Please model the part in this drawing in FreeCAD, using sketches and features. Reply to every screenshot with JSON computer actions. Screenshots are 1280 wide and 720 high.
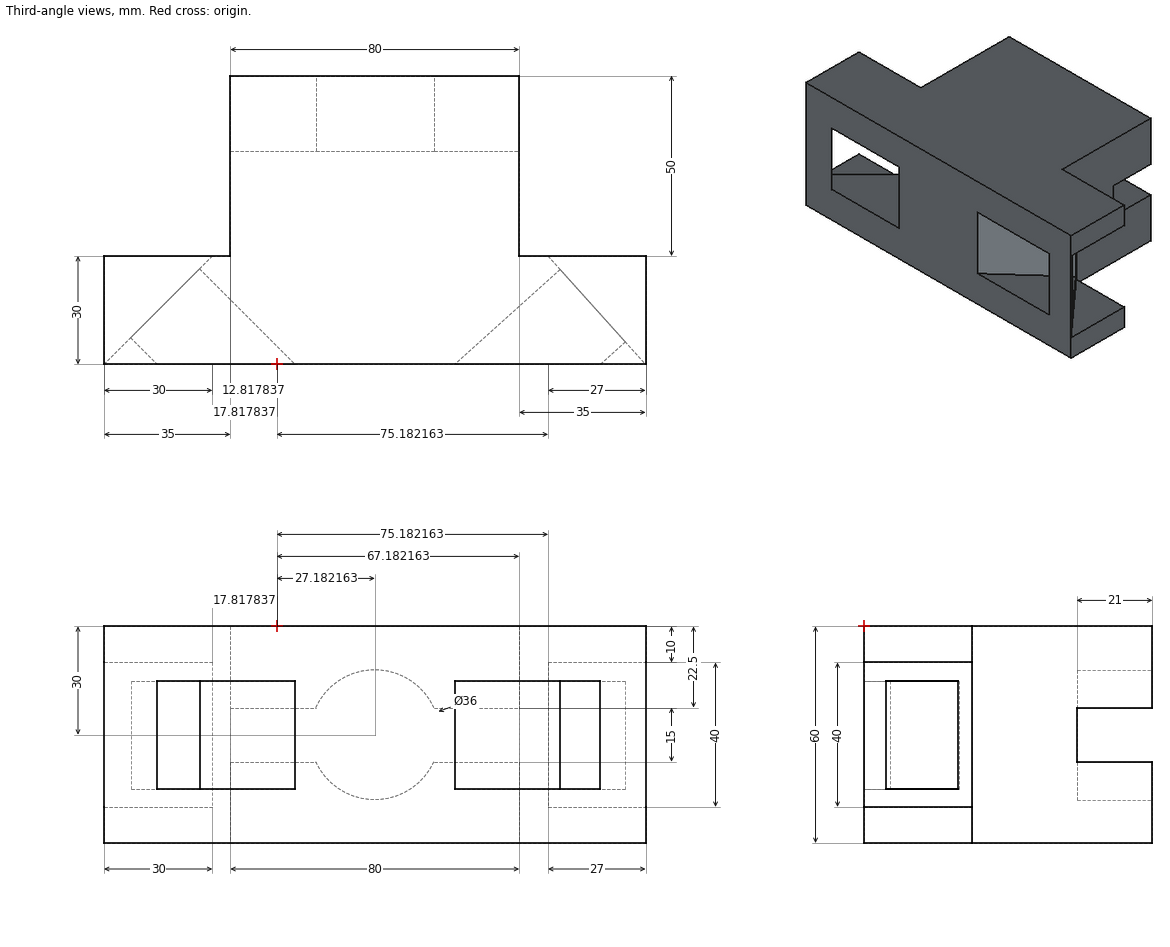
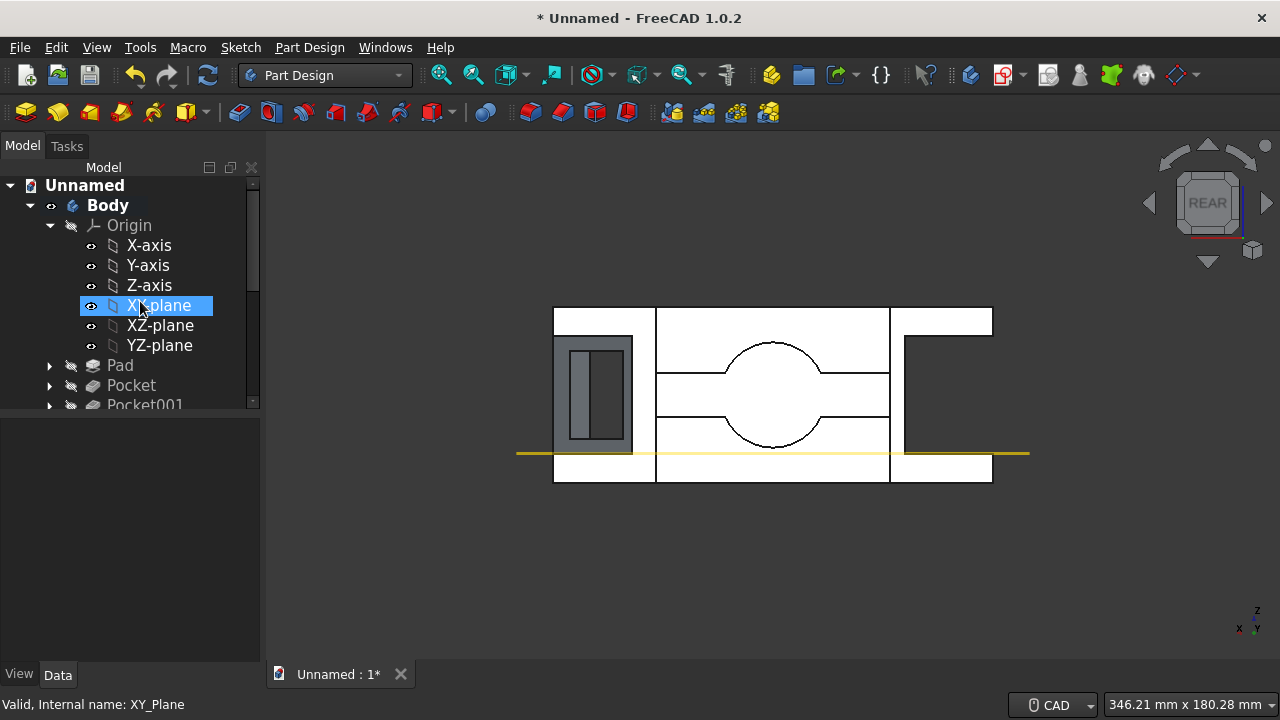
{"action": "scroll", "coordinate": [100, 301], "scroll_direction": "down", "scroll_amount": 6}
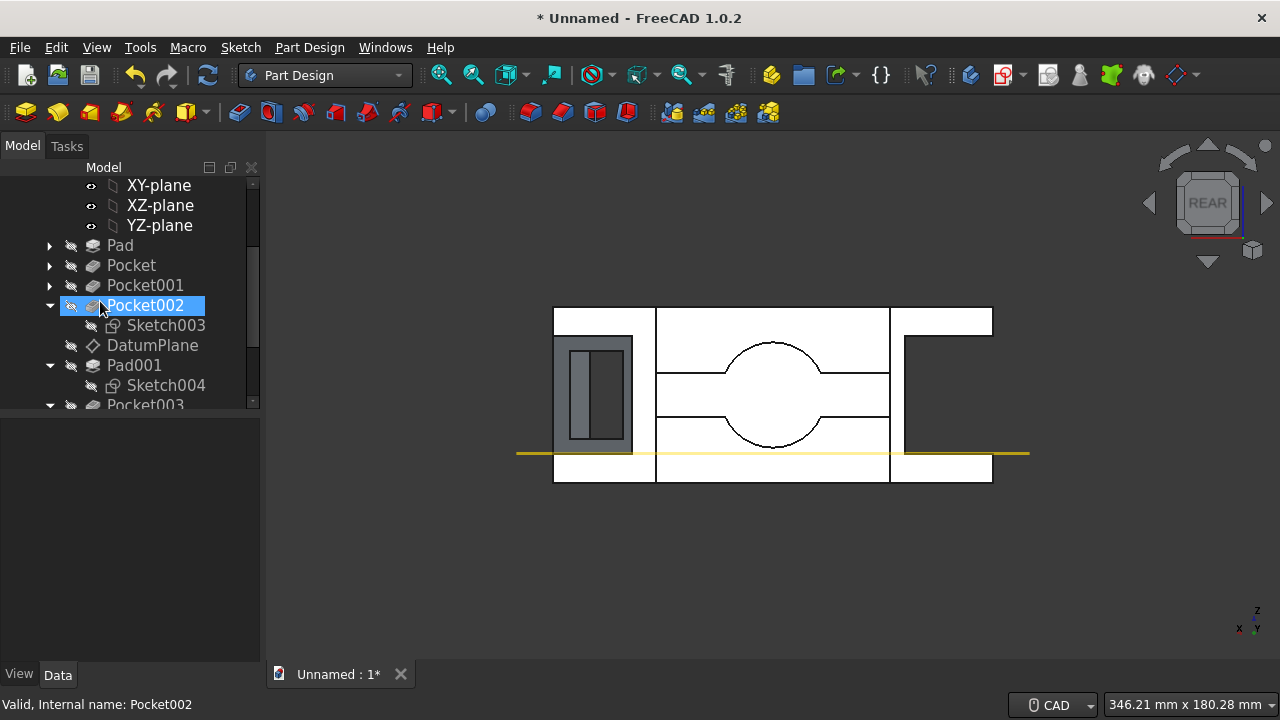
{"action": "left_click", "coordinate": [116, 386]}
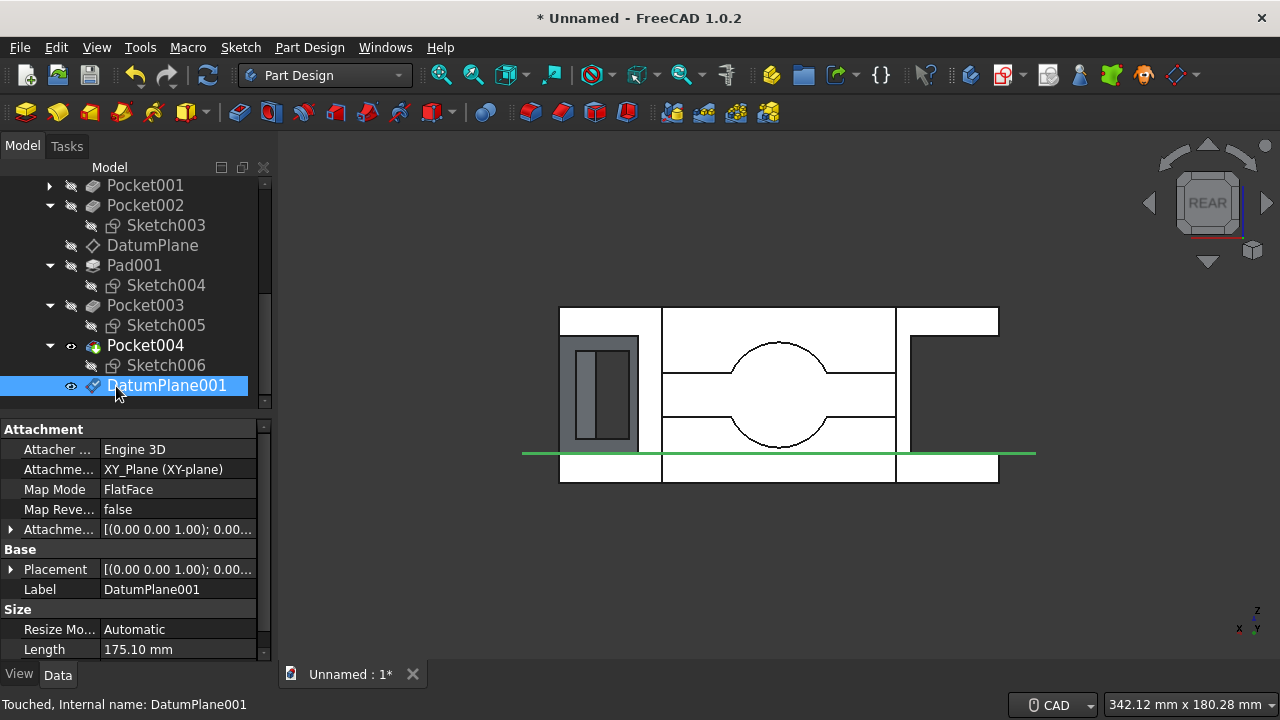
{"action": "left_click", "coordinate": [1004, 76]}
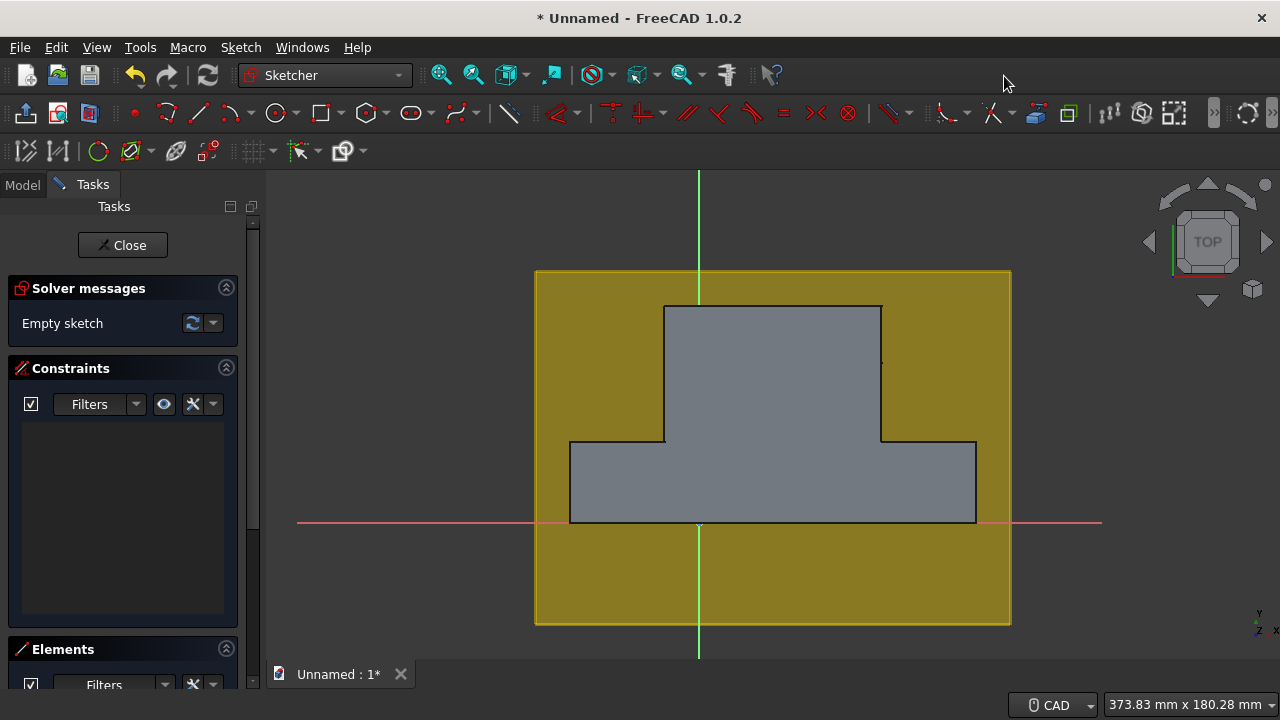
{"action": "left_click", "coordinate": [90, 114]}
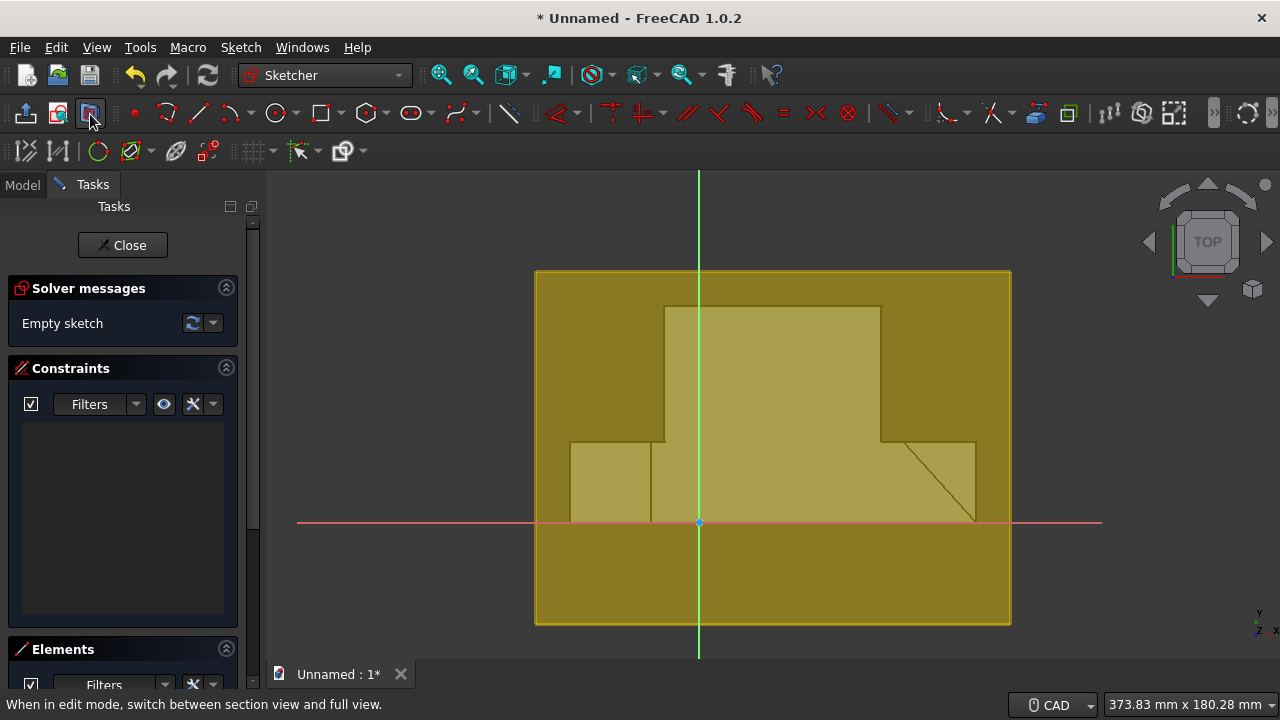
{"action": "scroll", "coordinate": [611, 505], "scroll_direction": "up", "scroll_amount": 7}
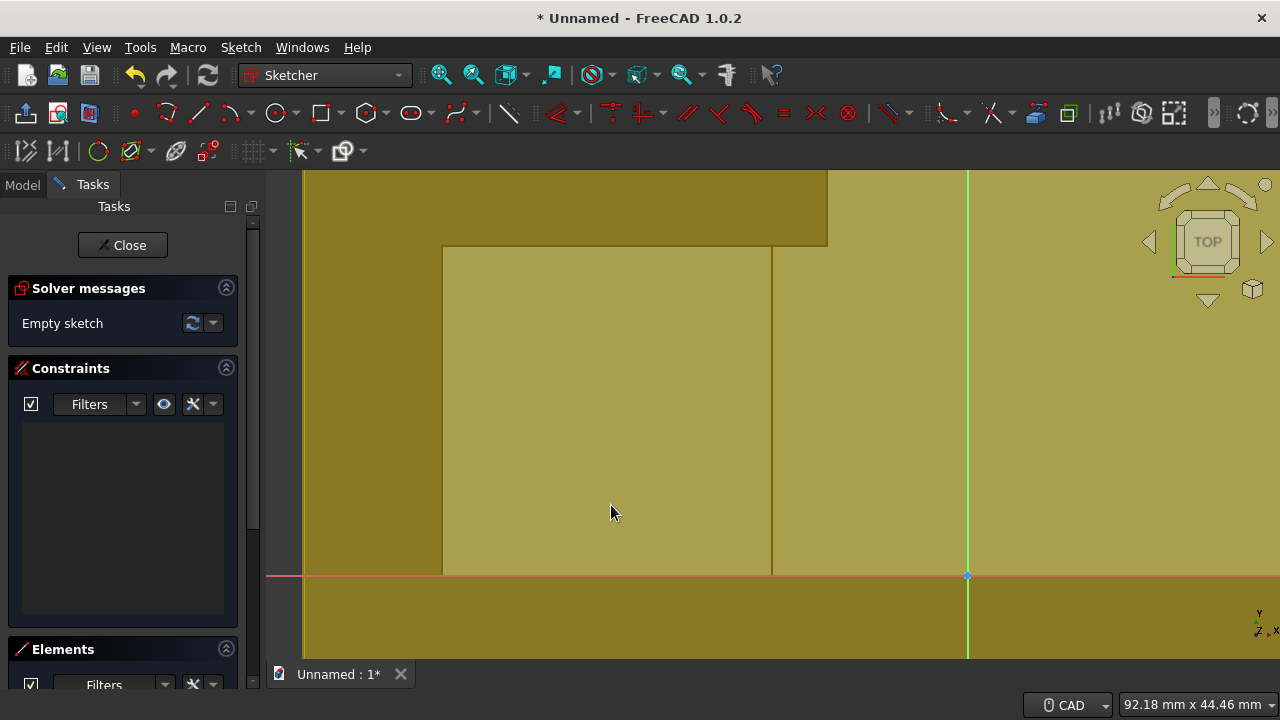
{"action": "left_click", "coordinate": [168, 114]}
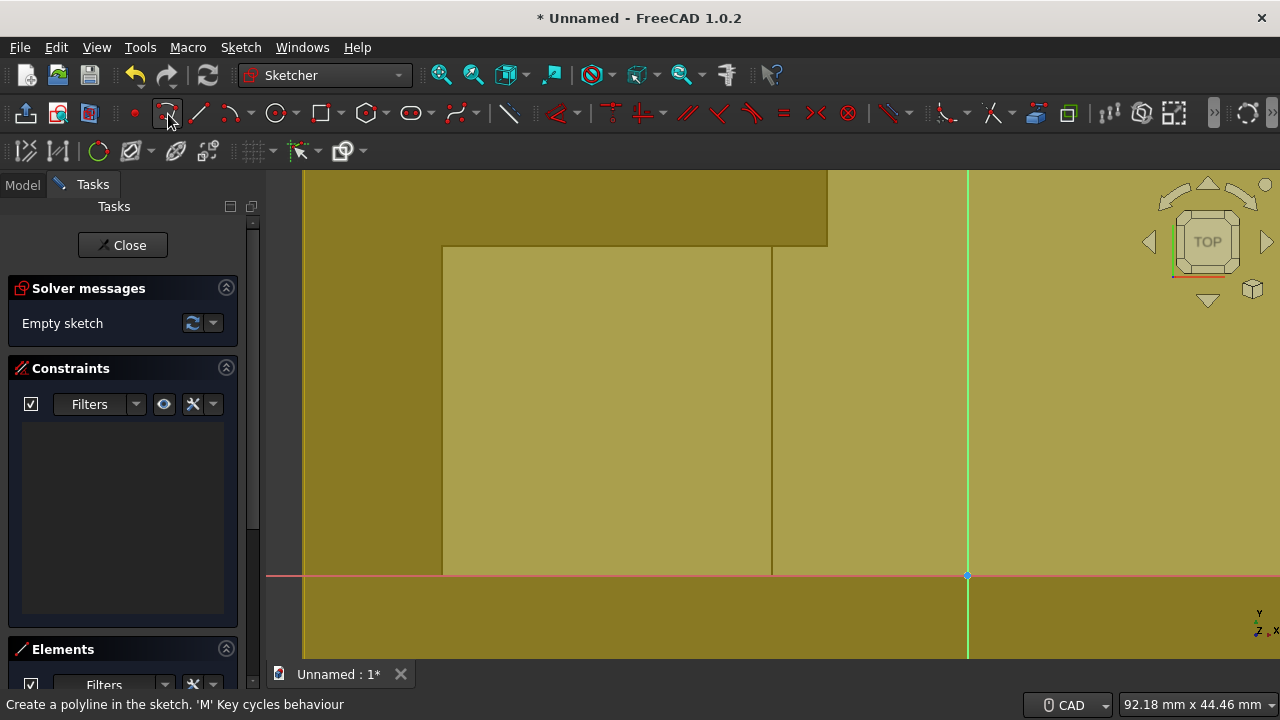
{"action": "left_click", "coordinate": [772, 576]}
{"action": "left_click", "coordinate": [772, 246]}
{"action": "left_click", "coordinate": [442, 567]}
{"action": "left_click", "coordinate": [772, 576]}
{"action": "key", "text": "Escape"}
{"action": "key", "text": "Escape"}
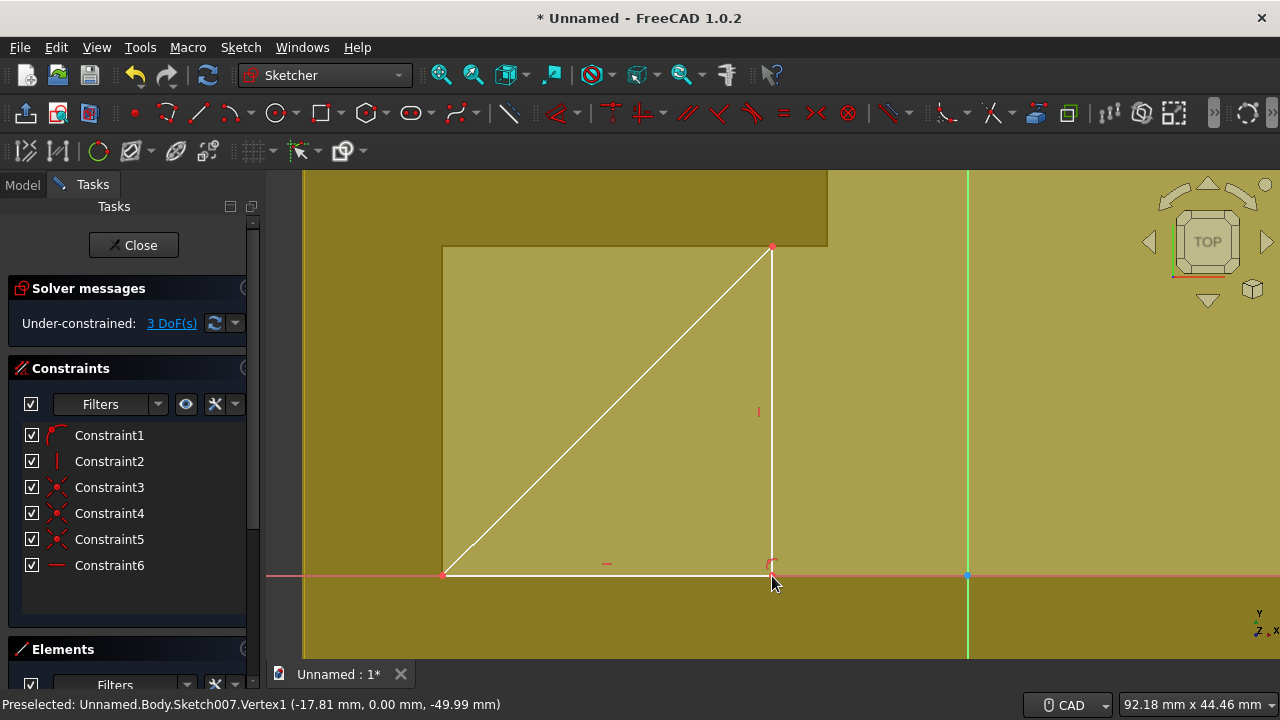
{"action": "left_click", "coordinate": [556, 114]}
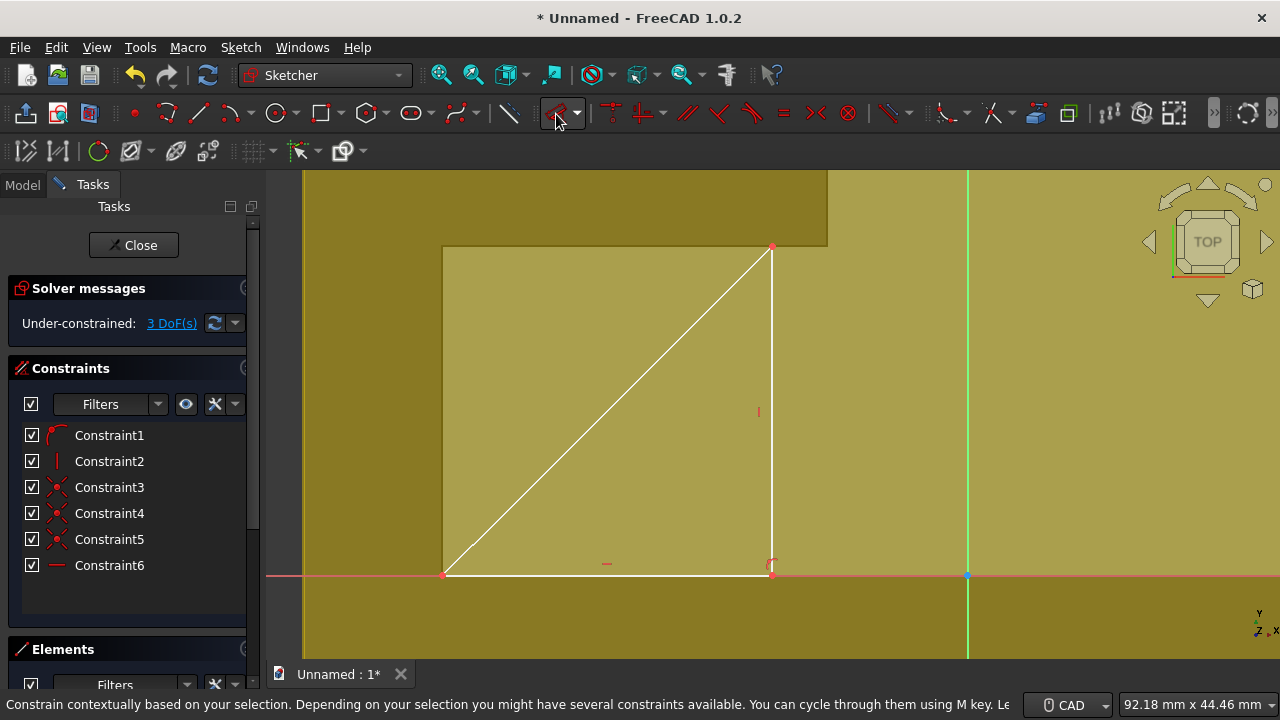
{"action": "left_click", "coordinate": [772, 477]}
{"action": "left_click", "coordinate": [806, 411]}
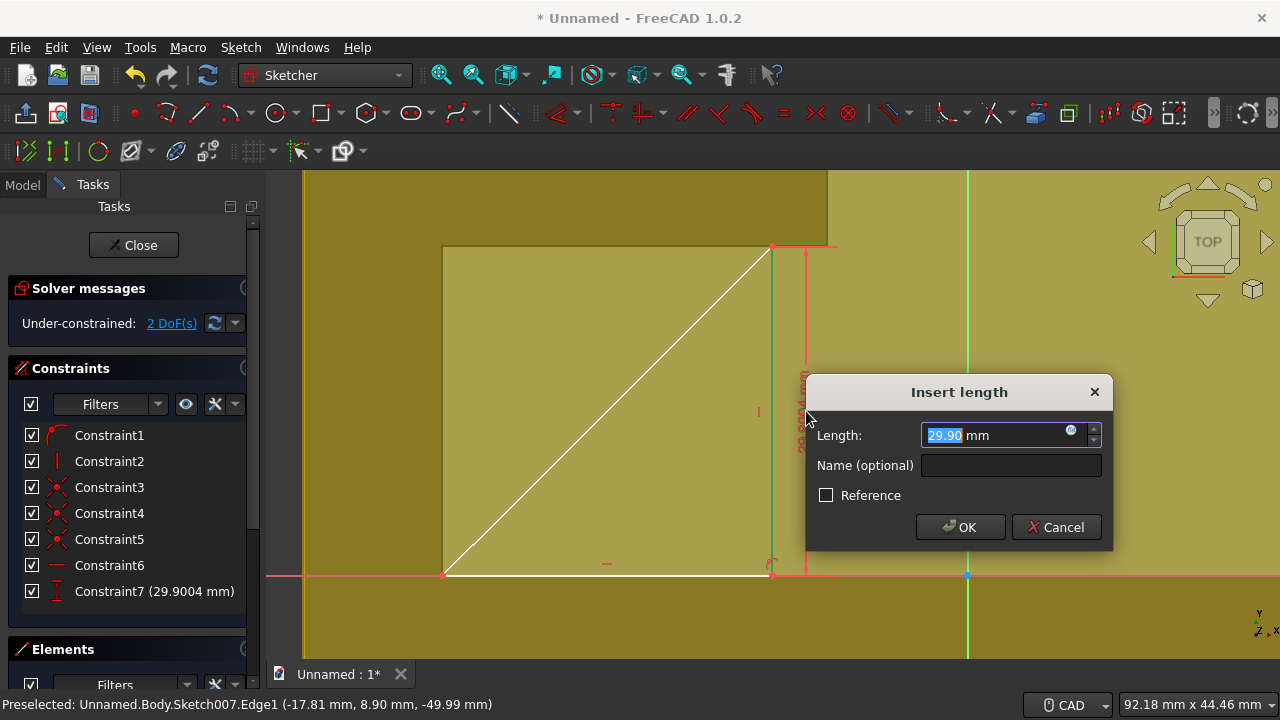
{"action": "type", "text": "30"}
{"action": "key", "text": "Return"}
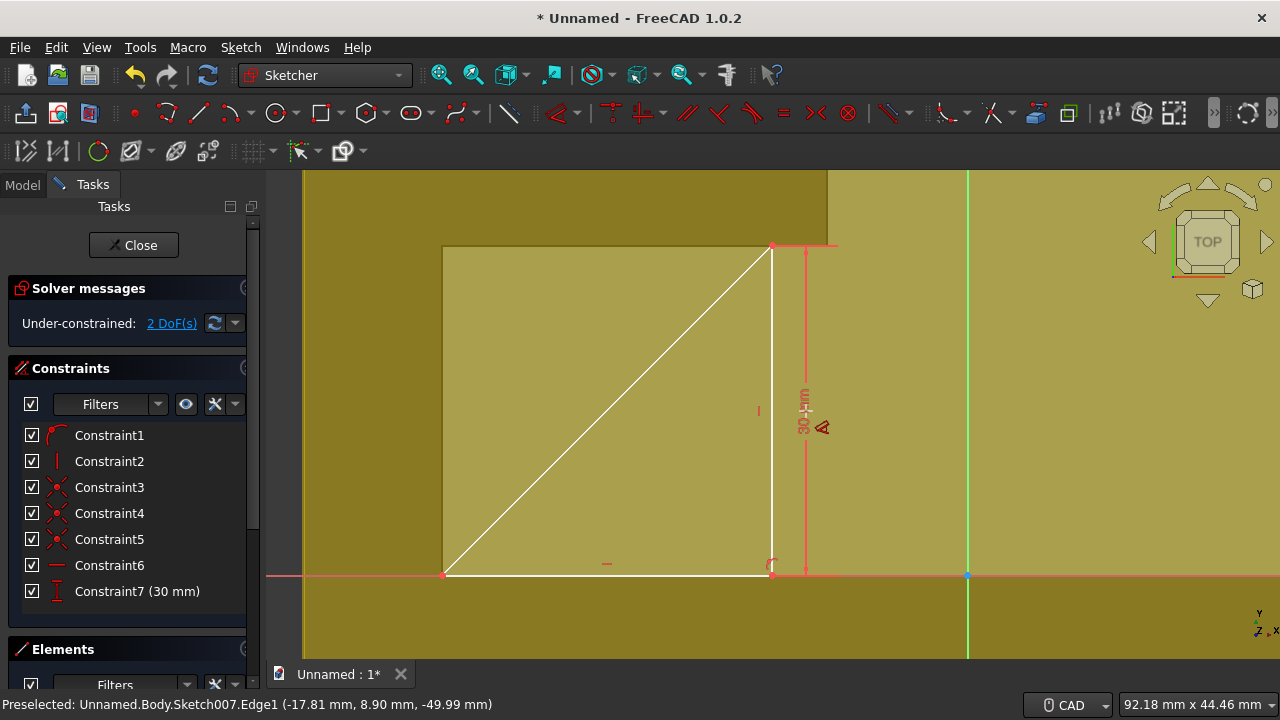
{"action": "left_click", "coordinate": [541, 576]}
{"action": "left_click", "coordinate": [607, 610]}